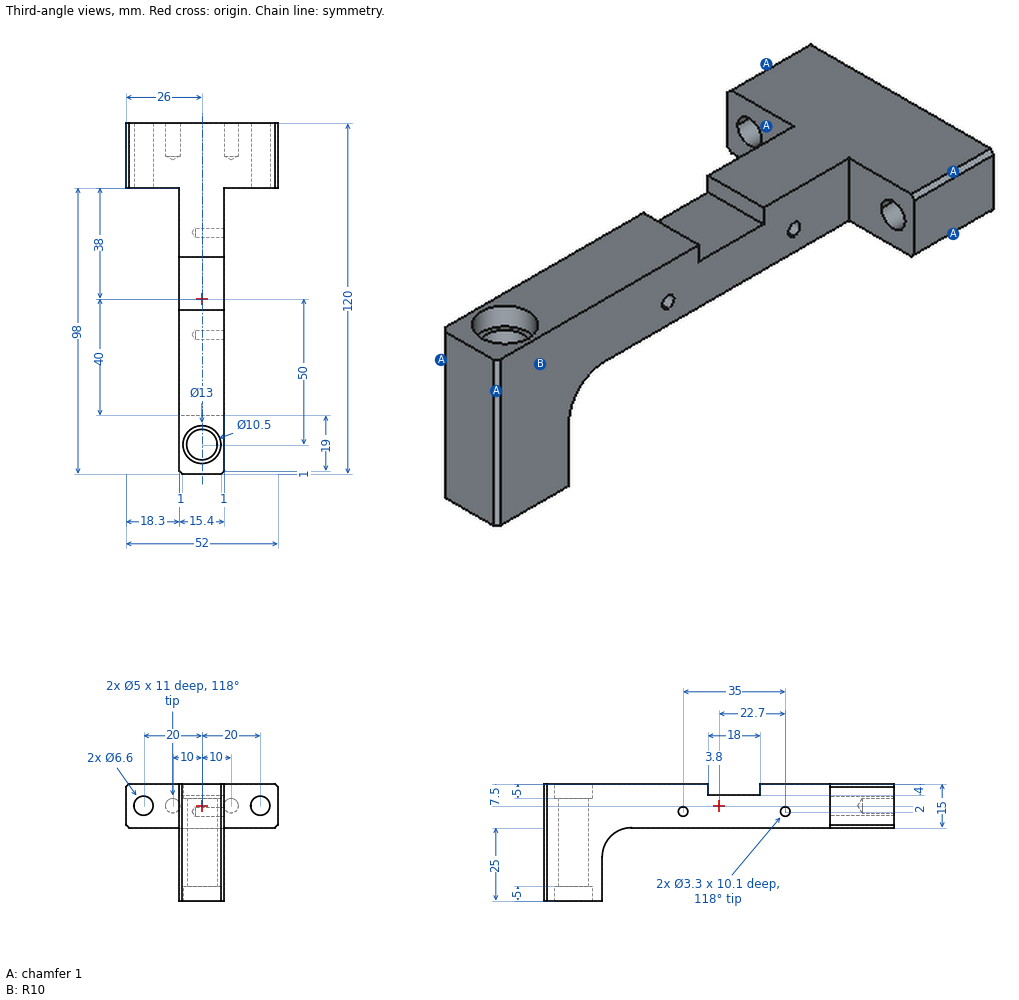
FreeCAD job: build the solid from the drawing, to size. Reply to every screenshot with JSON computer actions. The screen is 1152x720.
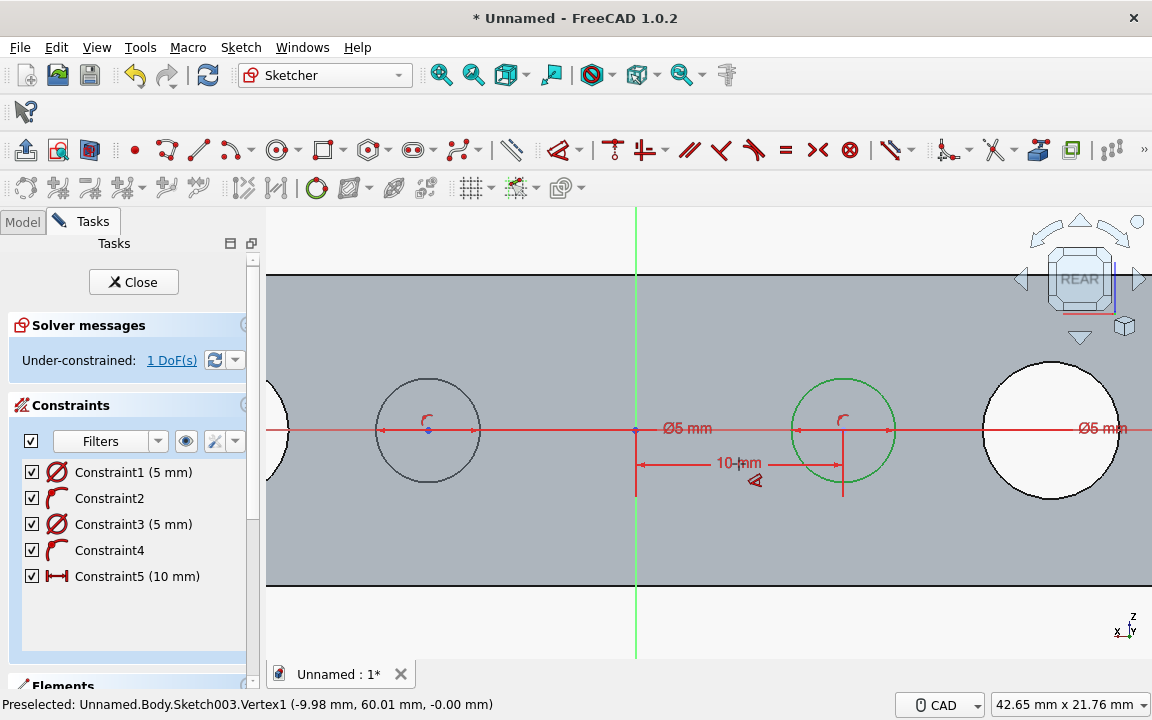
{"action": "left_click", "coordinate": [428, 430]}
{"action": "left_click", "coordinate": [532, 464]}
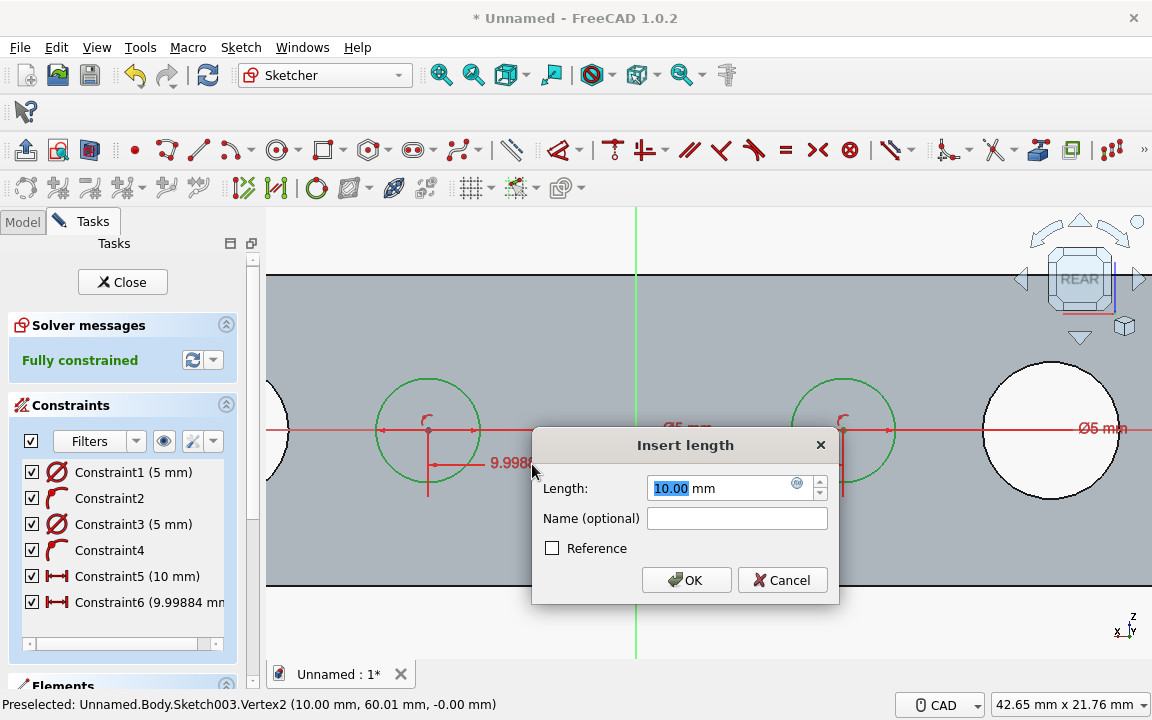
{"action": "type", "text": "10"}
{"action": "key", "text": "Return"}
{"action": "key", "text": "Escape"}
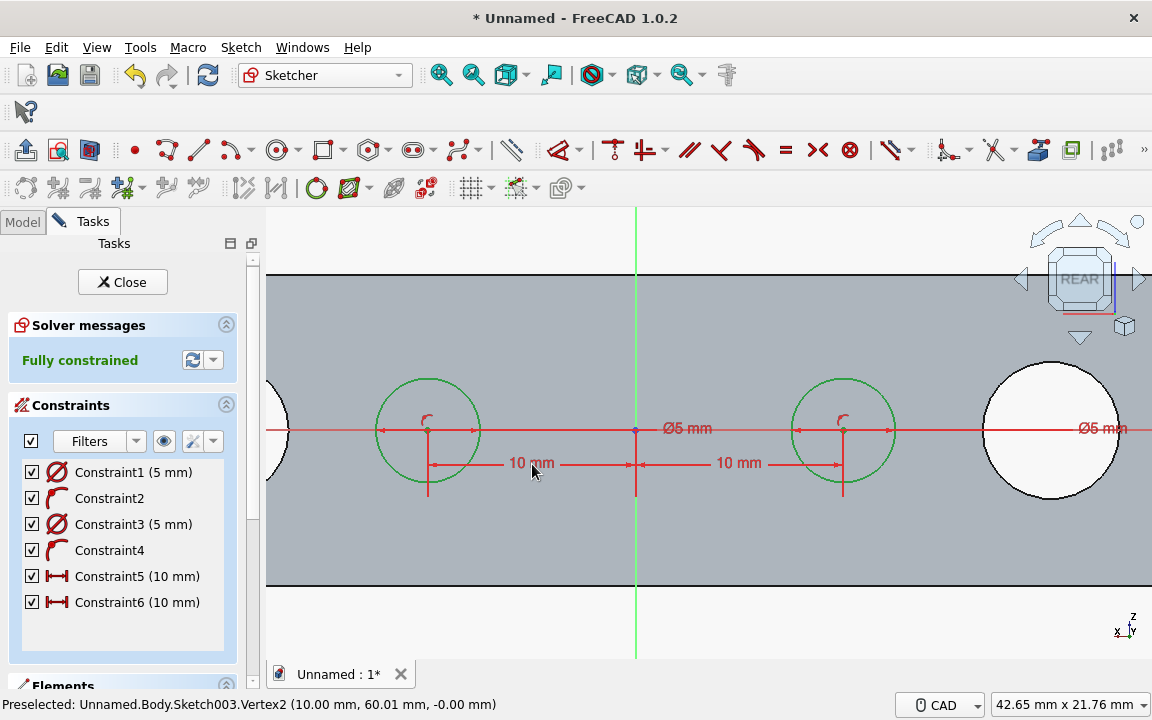
{"action": "left_click", "coordinate": [123, 282]}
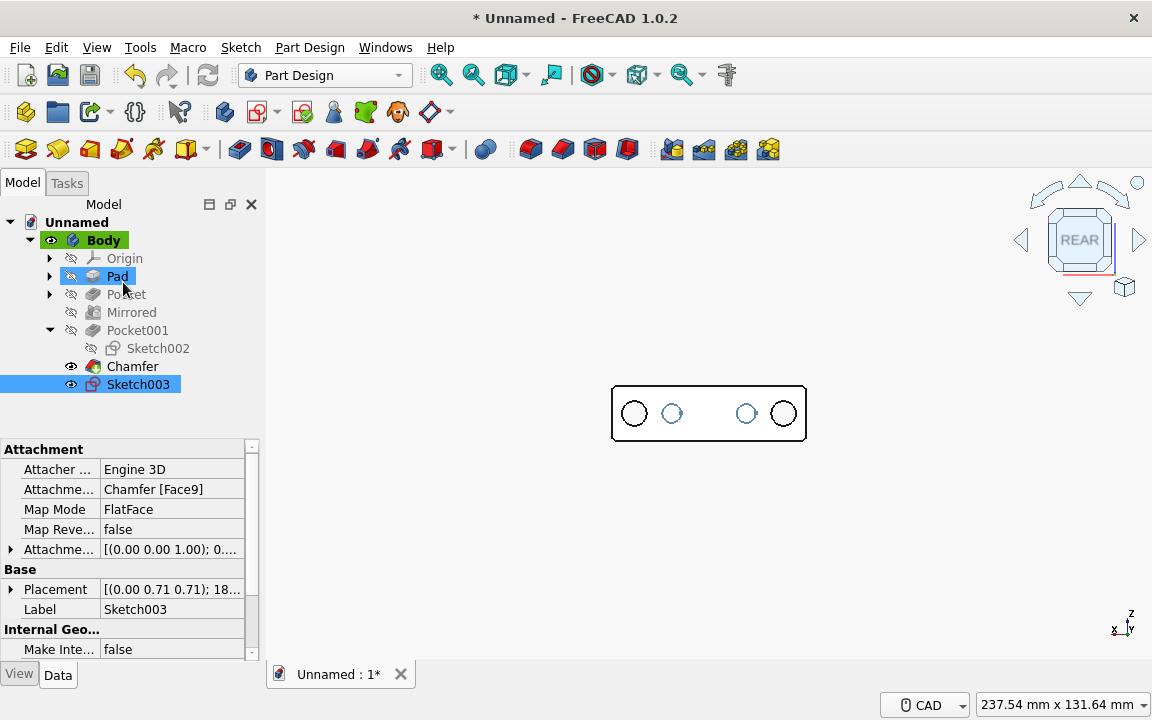
{"action": "left_click", "coordinate": [272, 150]}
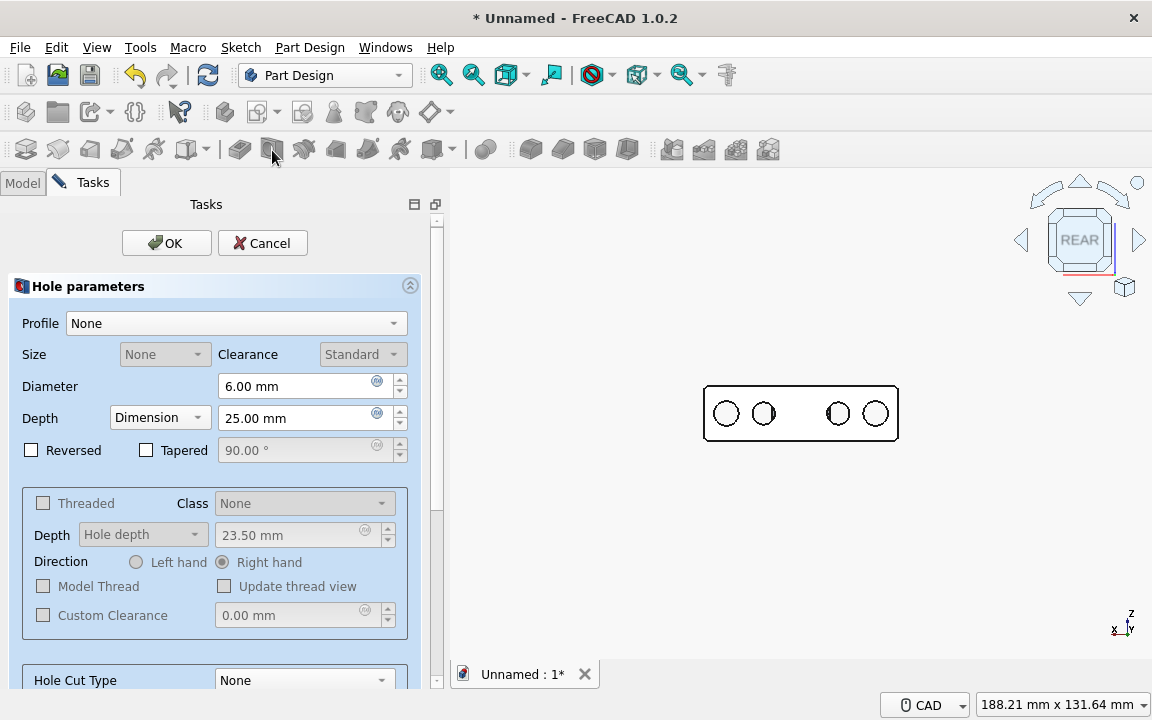
{"action": "triple_click", "coordinate": [305, 386]}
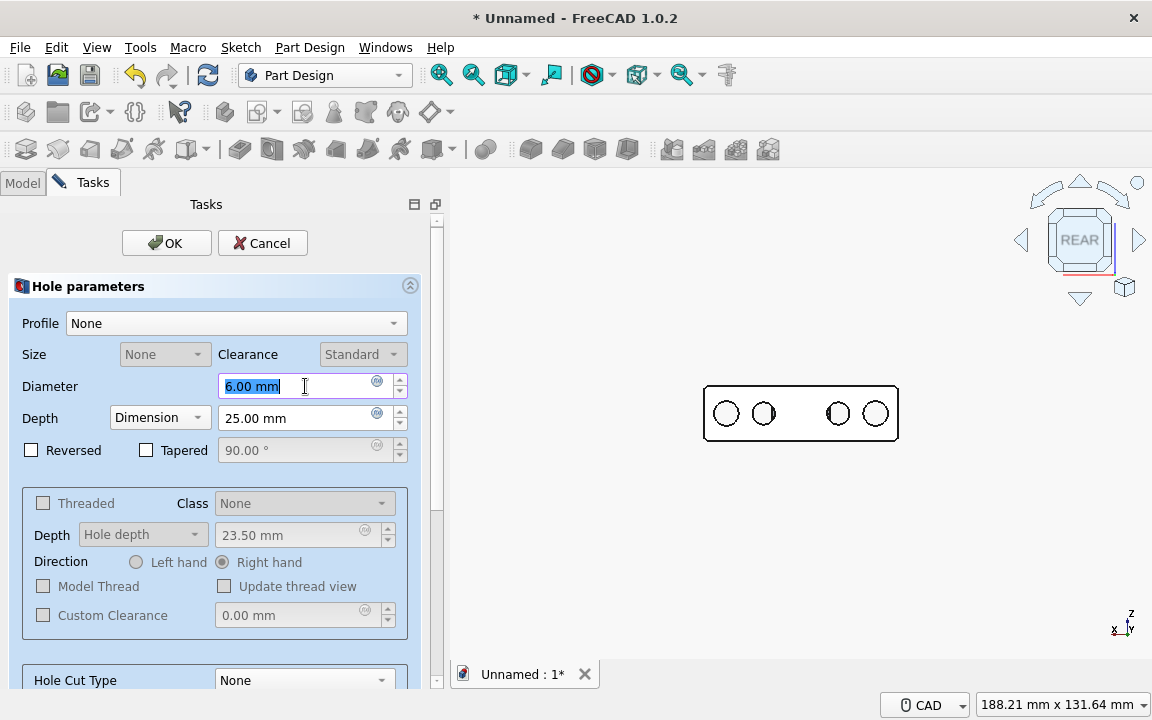
{"action": "type", "text": "5"}
{"action": "key", "text": "Tab"}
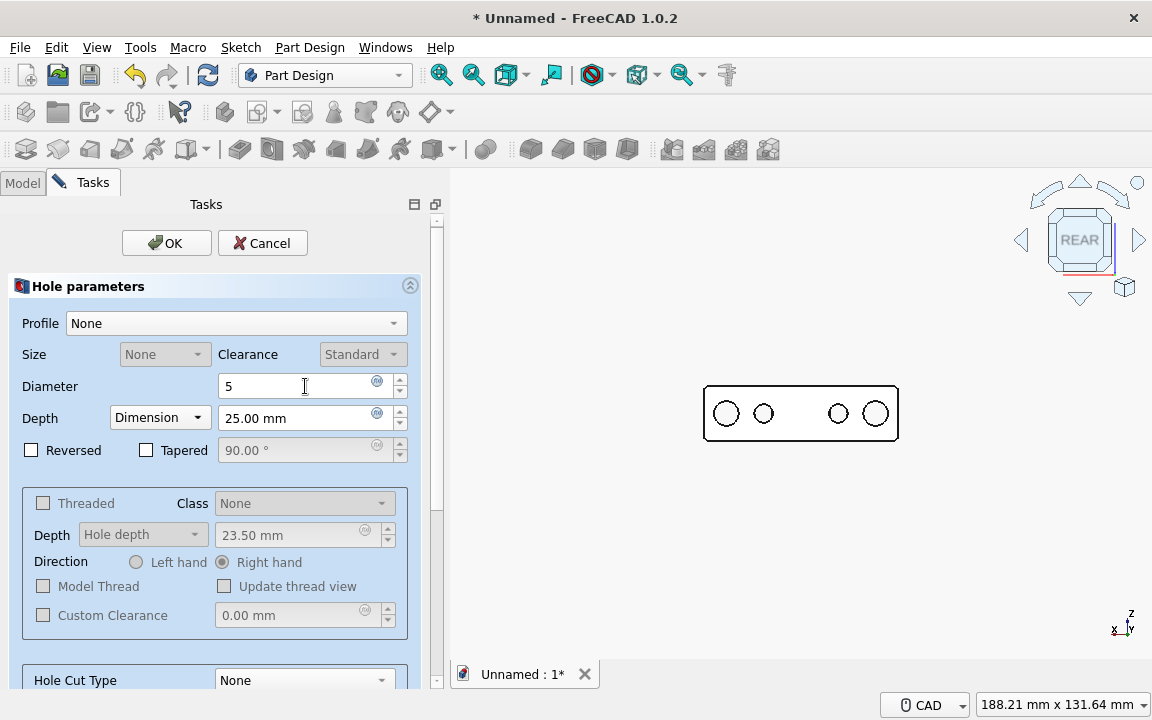
{"action": "triple_click", "coordinate": [305, 418]}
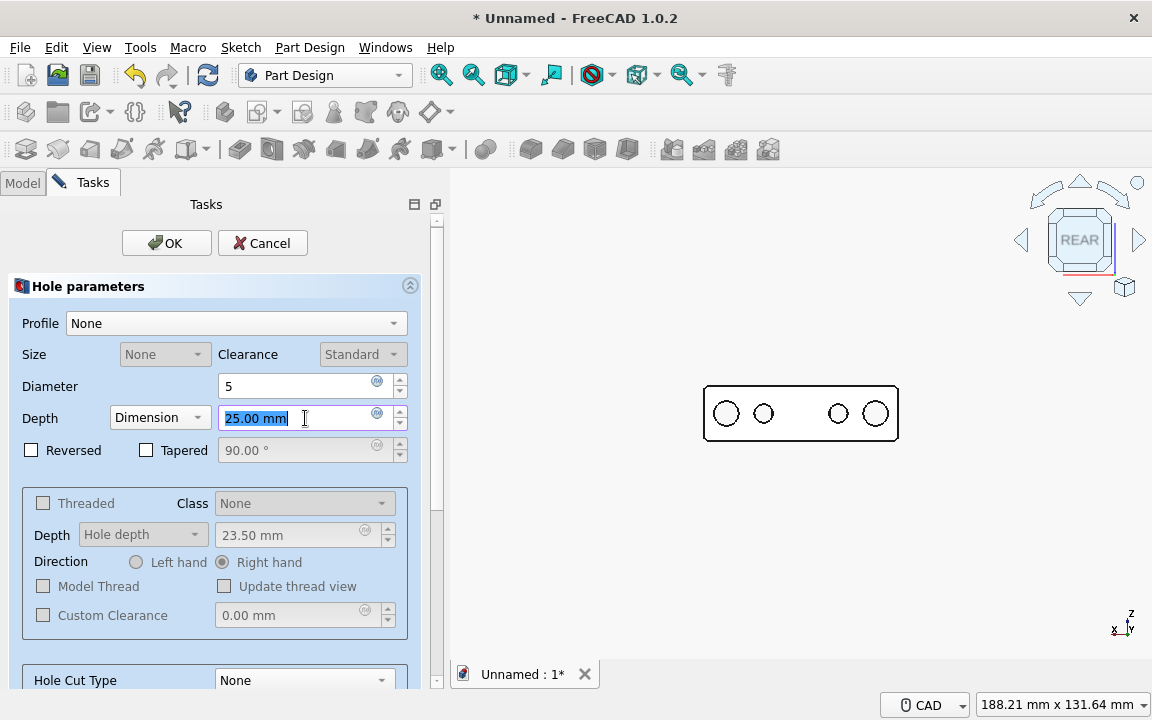
{"action": "type", "text": "11"}
{"action": "key", "text": "Tab"}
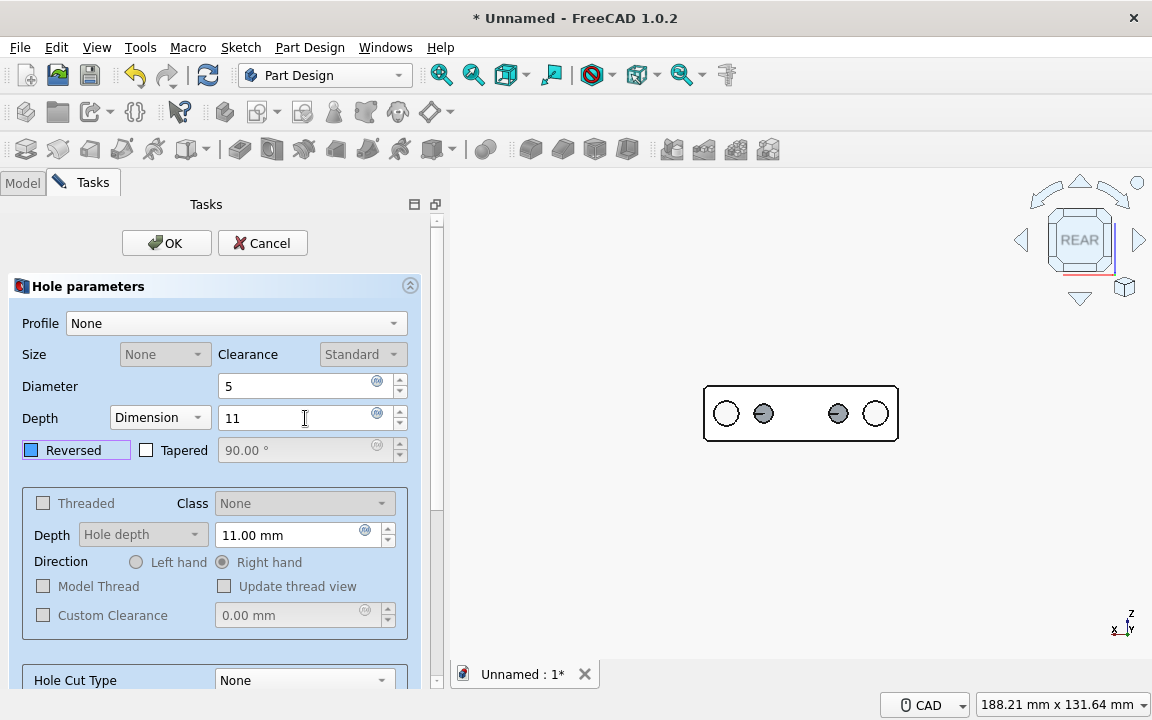
{"action": "left_click", "coordinate": [167, 243]}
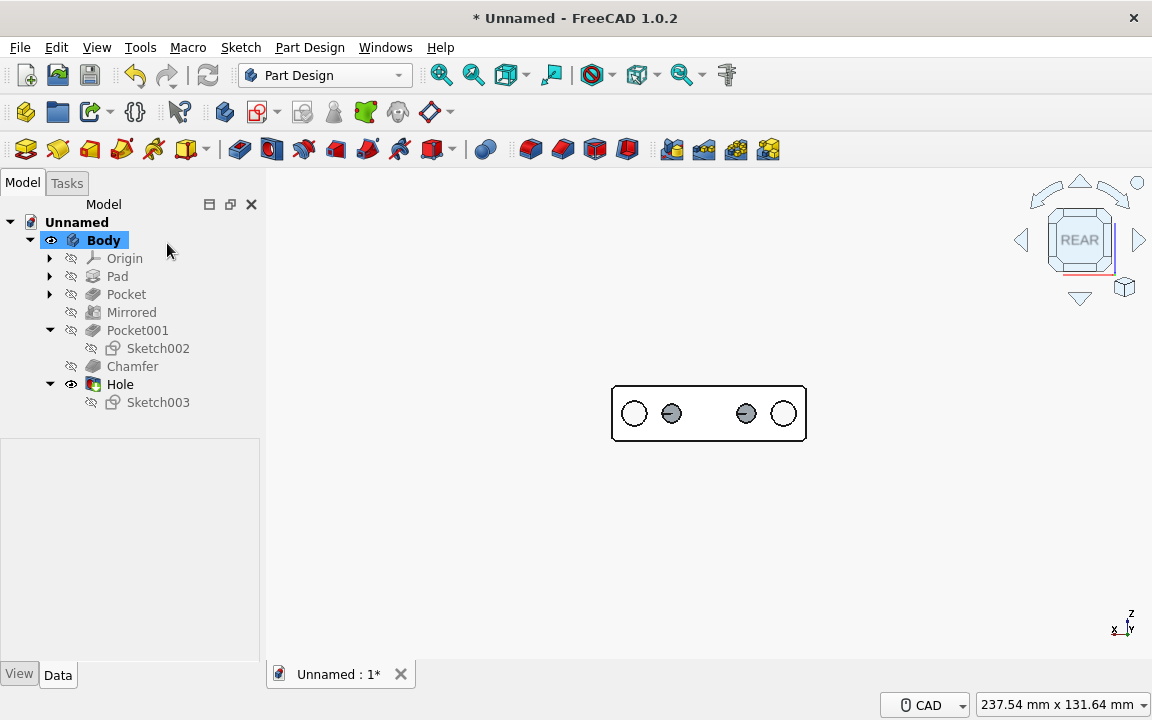
{"action": "left_click", "coordinate": [442, 76]}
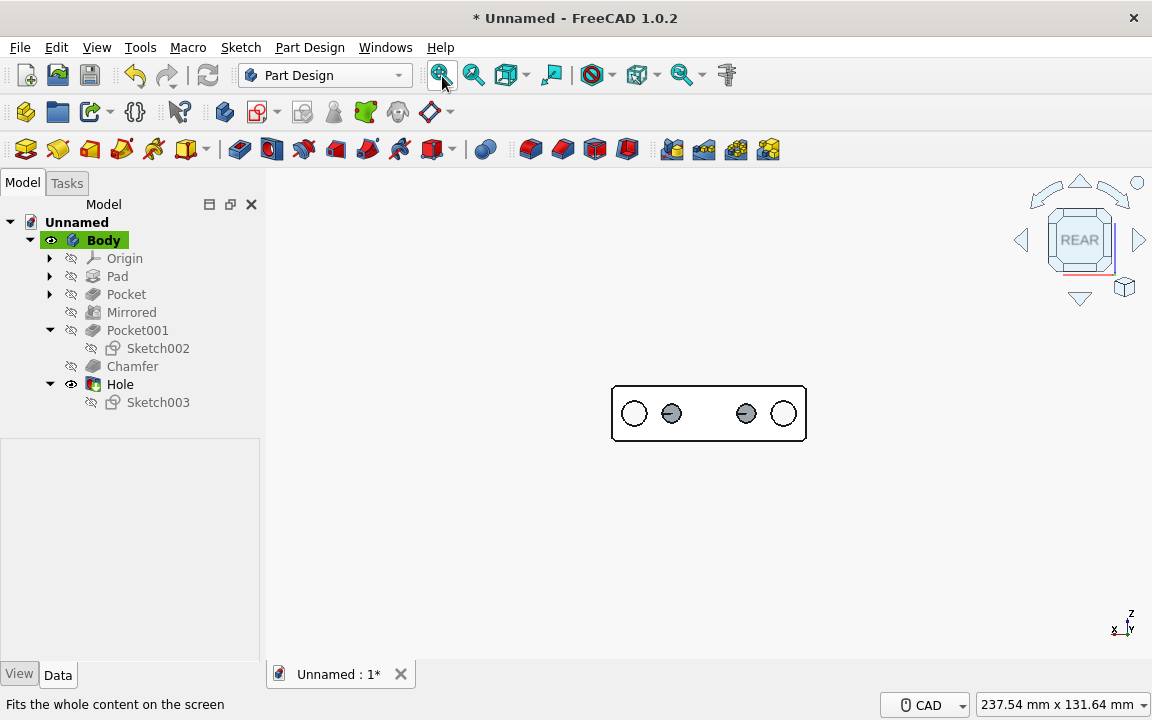
{"action": "key", "text": "5"}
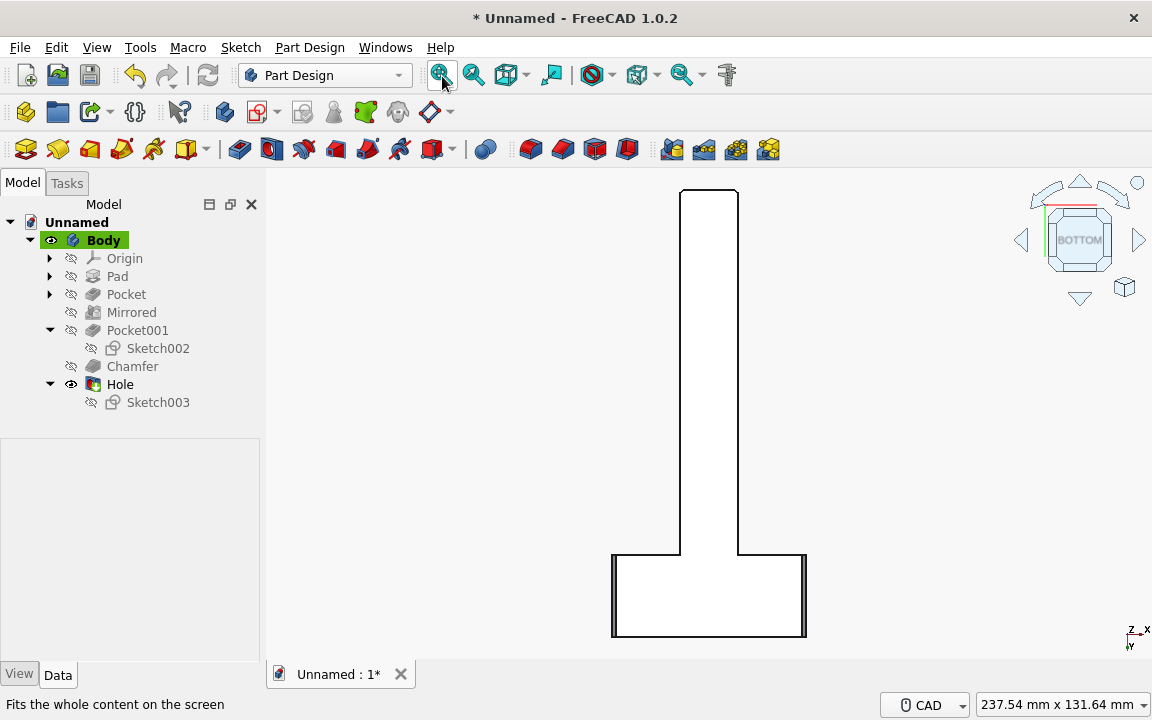
{"action": "left_click", "coordinate": [762, 604]}